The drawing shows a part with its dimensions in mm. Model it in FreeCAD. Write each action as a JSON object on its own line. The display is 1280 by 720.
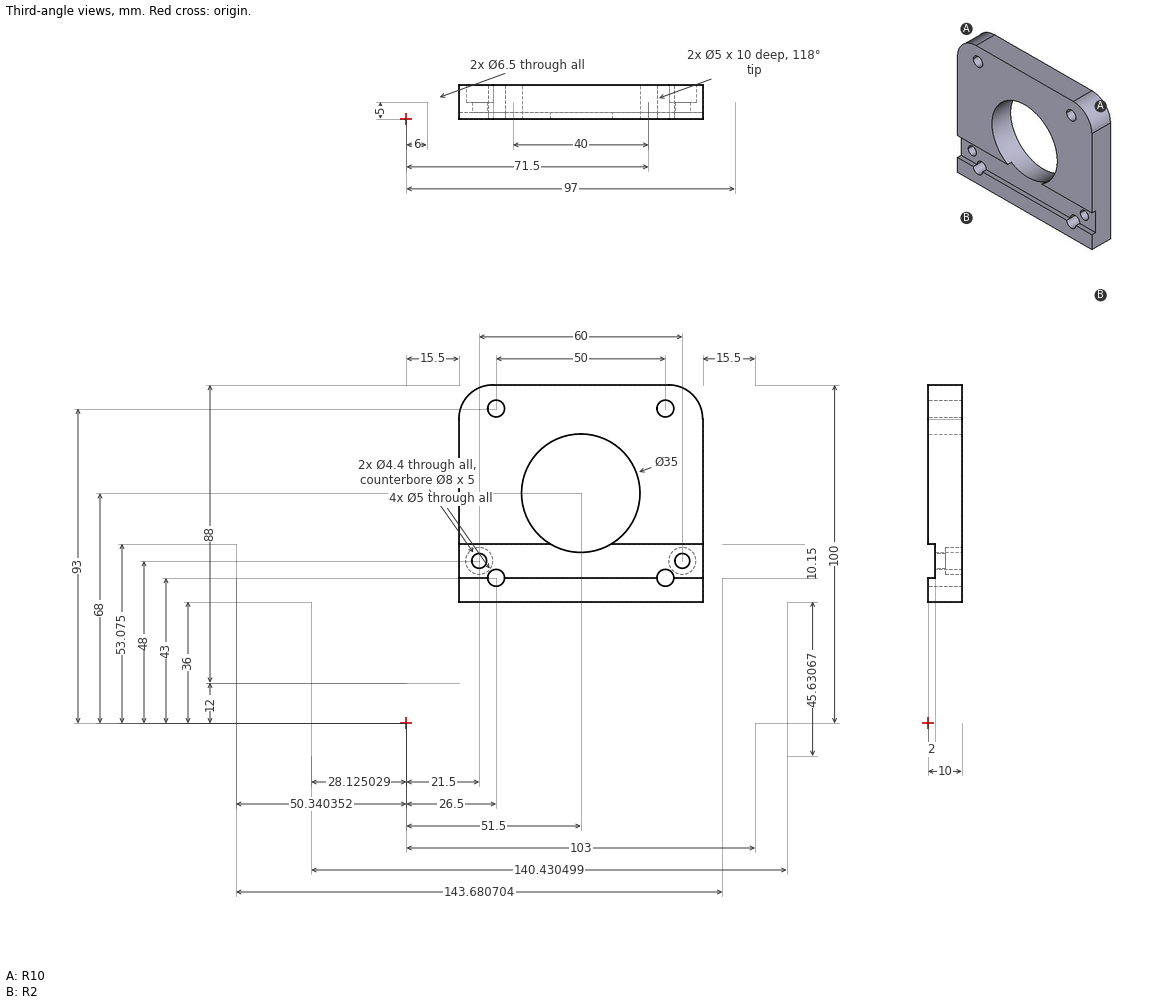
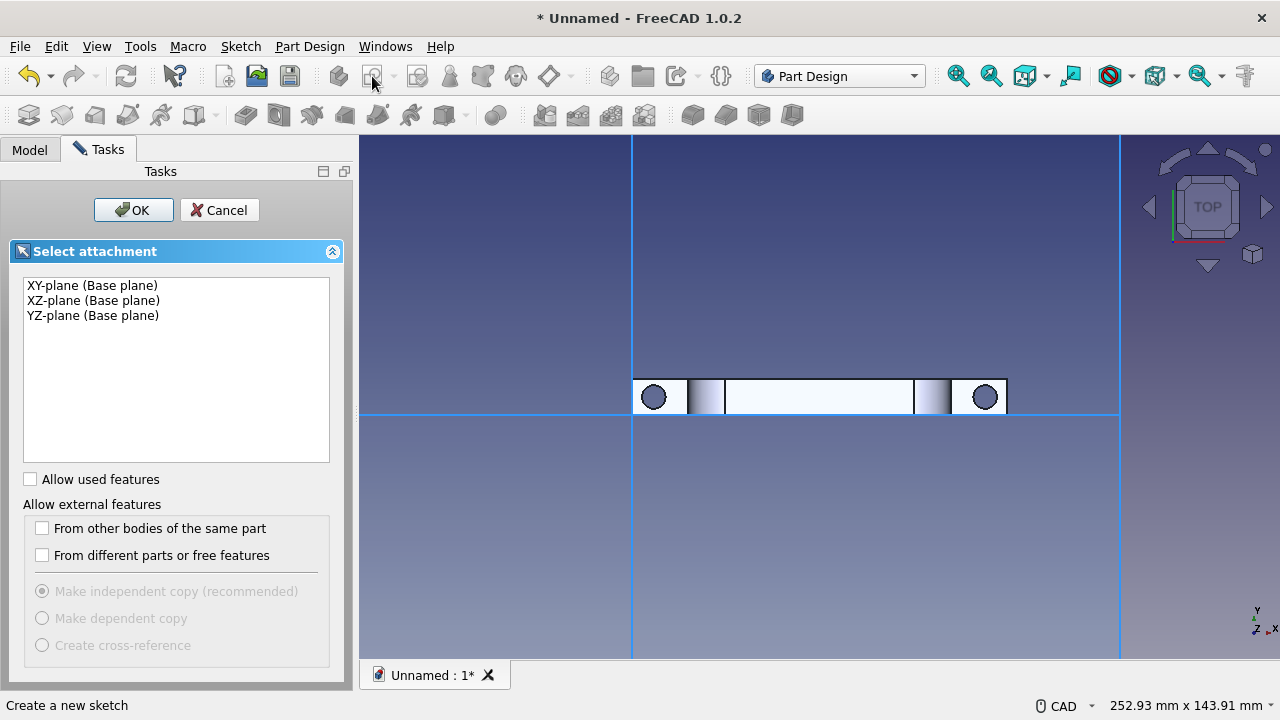
{"action": "left_click", "coordinate": [84, 286]}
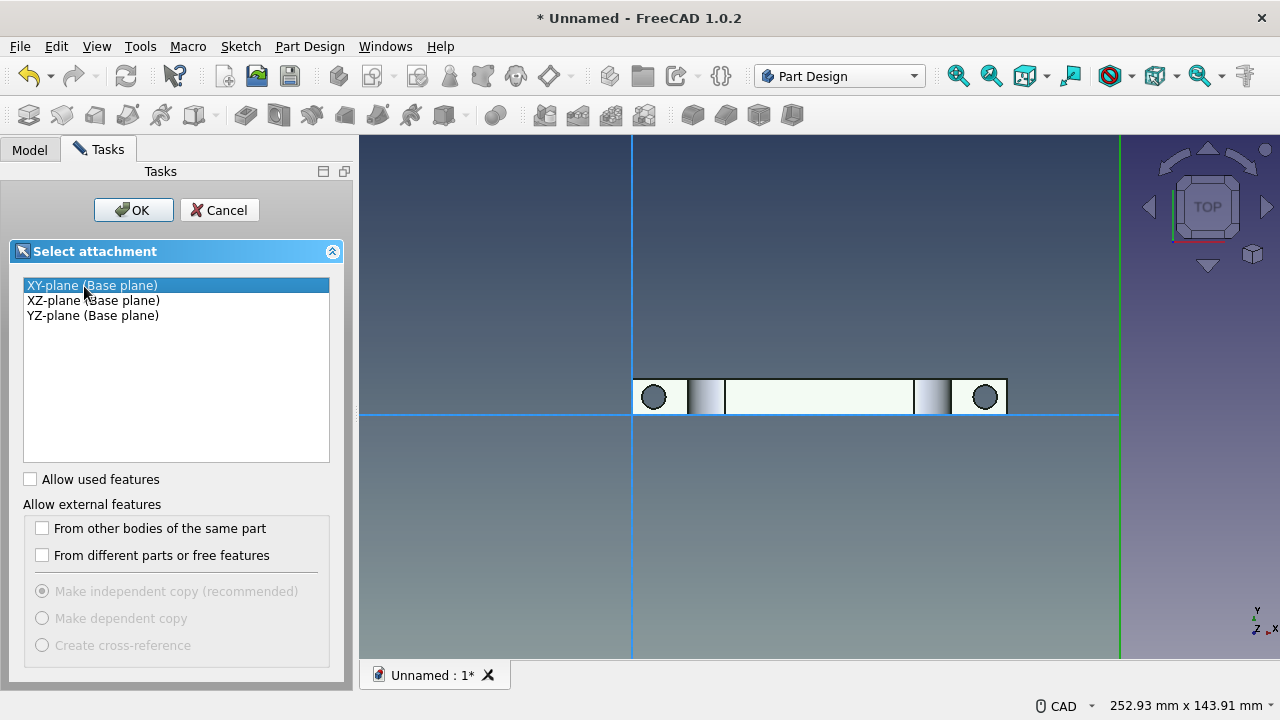
{"action": "left_click", "coordinate": [134, 210]}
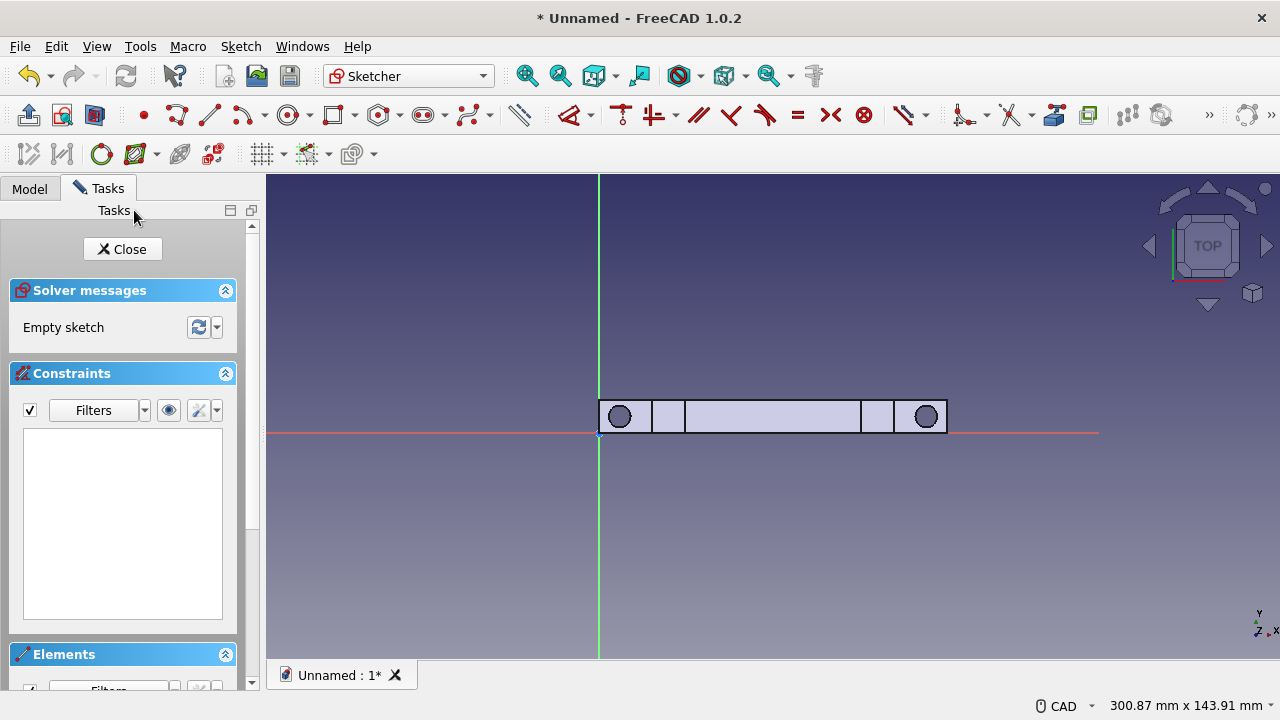
{"action": "left_click", "coordinate": [95, 116]}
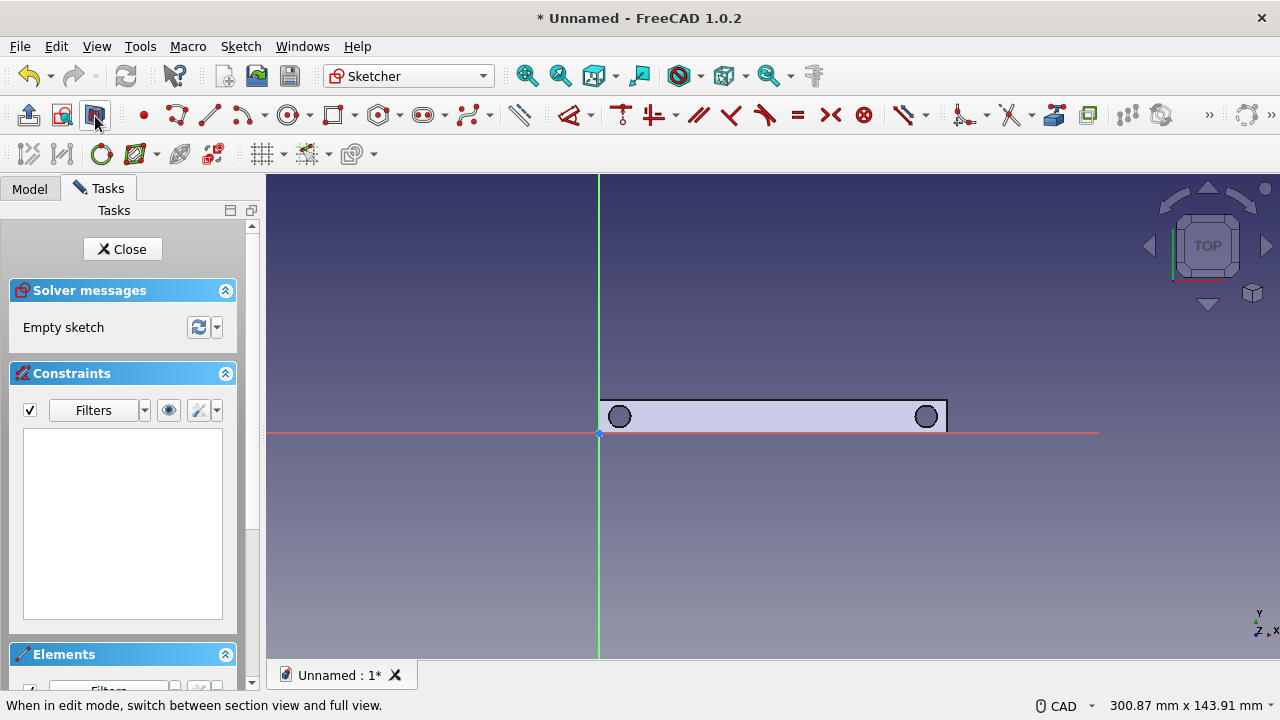
{"action": "scroll", "coordinate": [740, 424], "scroll_direction": "up", "scroll_amount": 4}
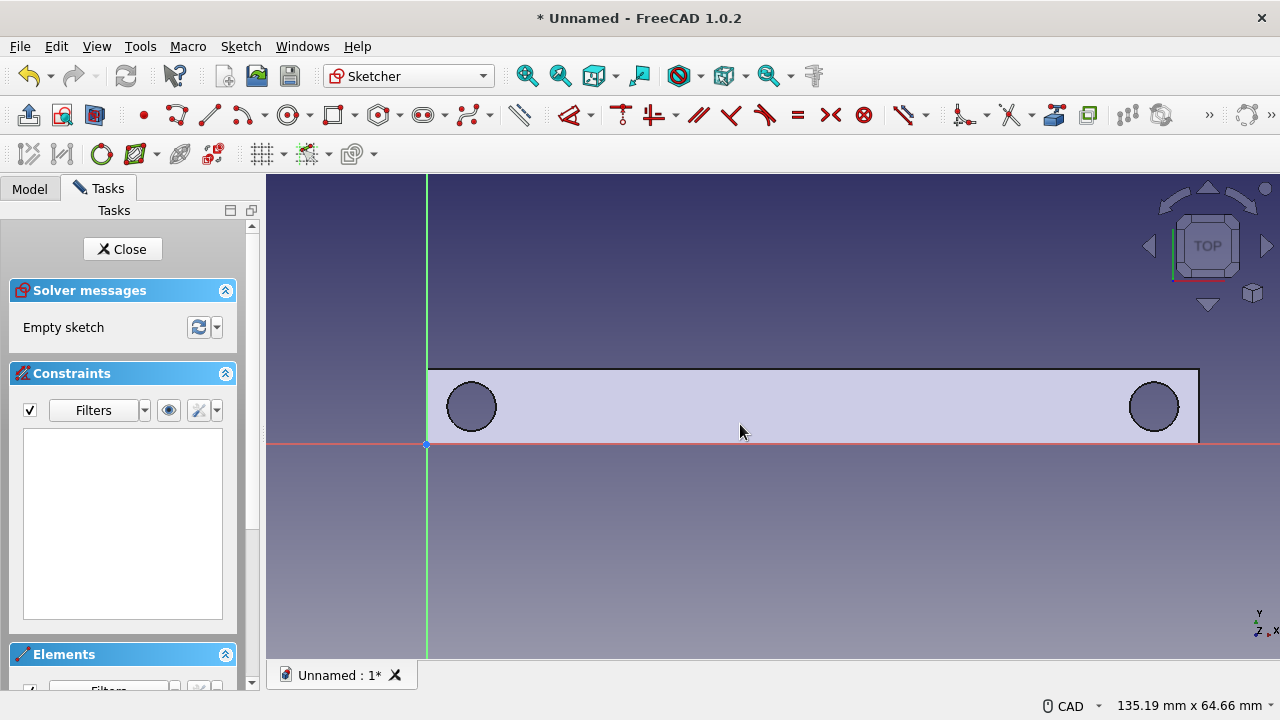
{"action": "left_click", "coordinate": [288, 116]}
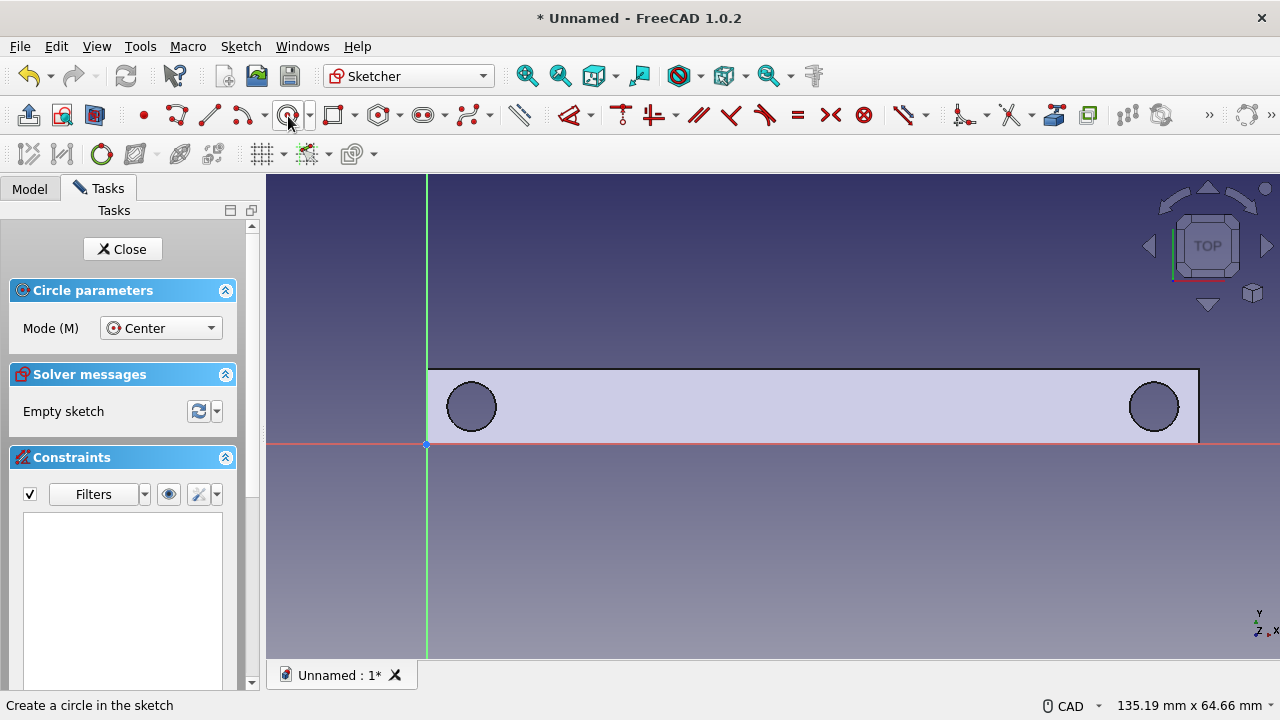
{"action": "left_click", "coordinate": [963, 407]}
{"action": "mouse_move", "coordinate": [976, 393]}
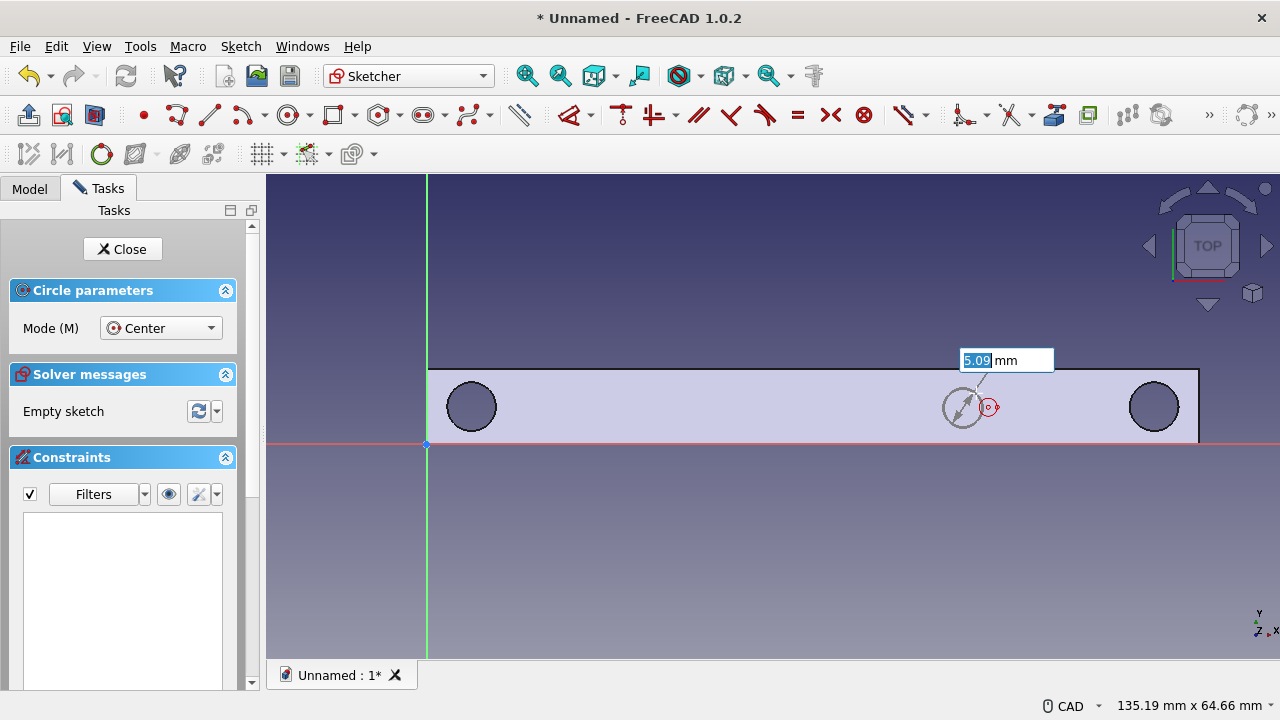
{"action": "type", "text": "5"}
{"action": "key", "text": "Return"}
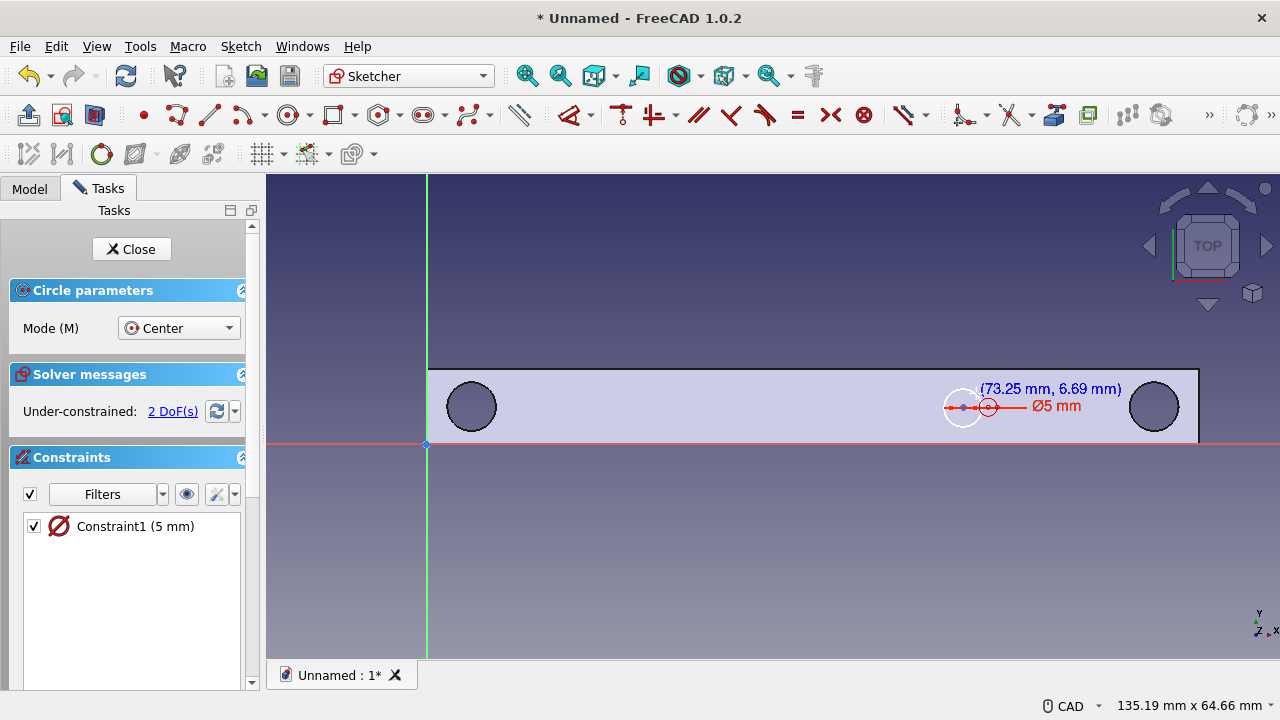
{"action": "left_click", "coordinate": [663, 407]}
{"action": "mouse_move", "coordinate": [676, 393]}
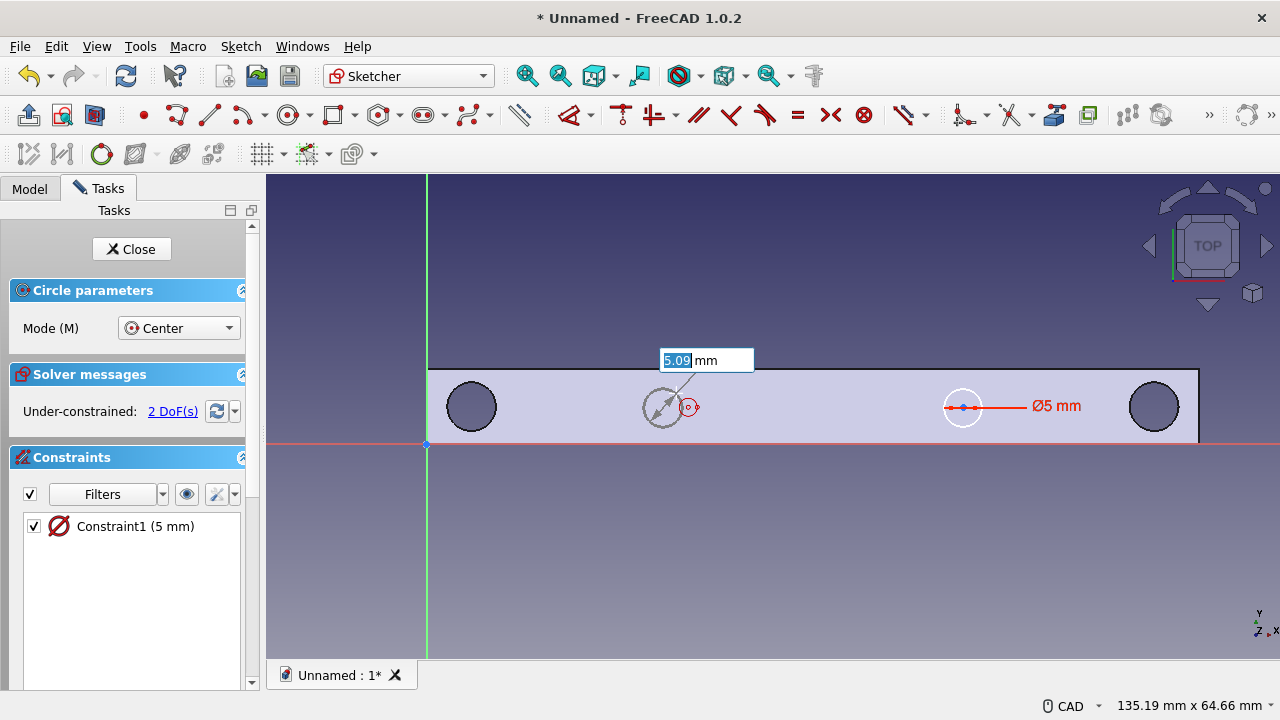
{"action": "type", "text": "5"}
{"action": "key", "text": "Return"}
{"action": "key", "text": "Escape"}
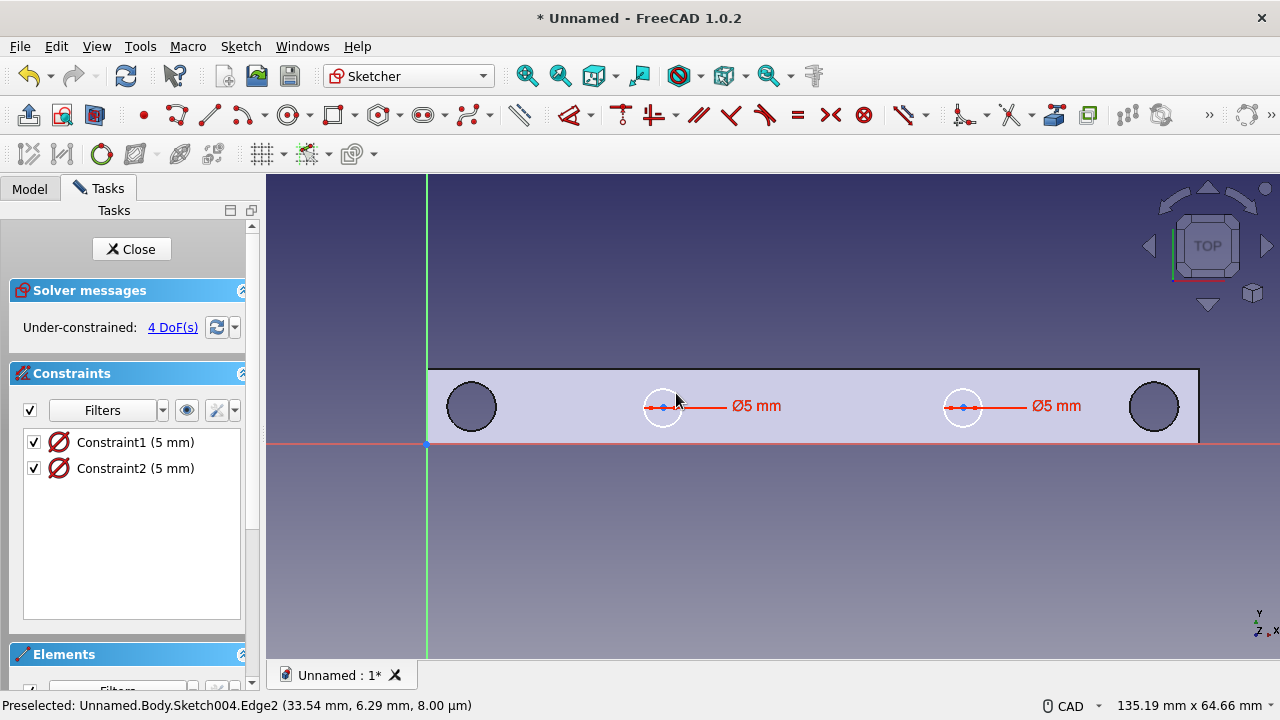
{"action": "key", "text": "d"}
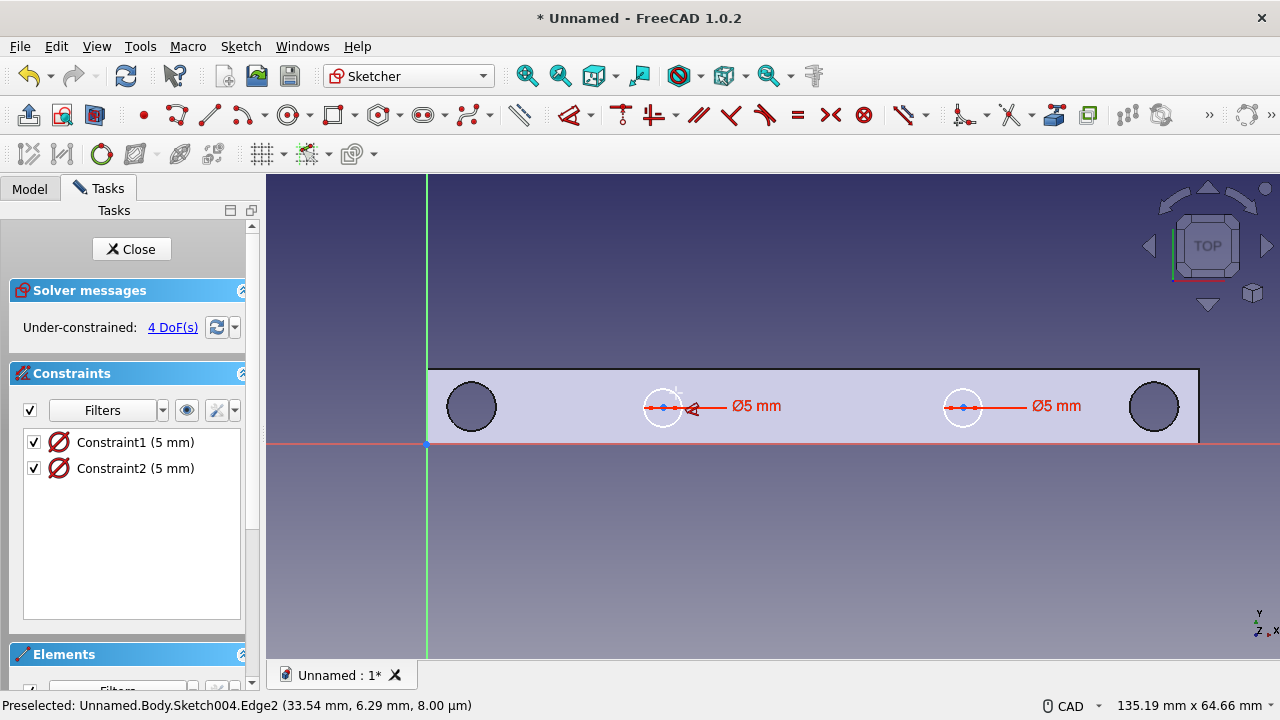
{"action": "left_click", "coordinate": [963, 408]}
{"action": "left_click", "coordinate": [393, 426]}